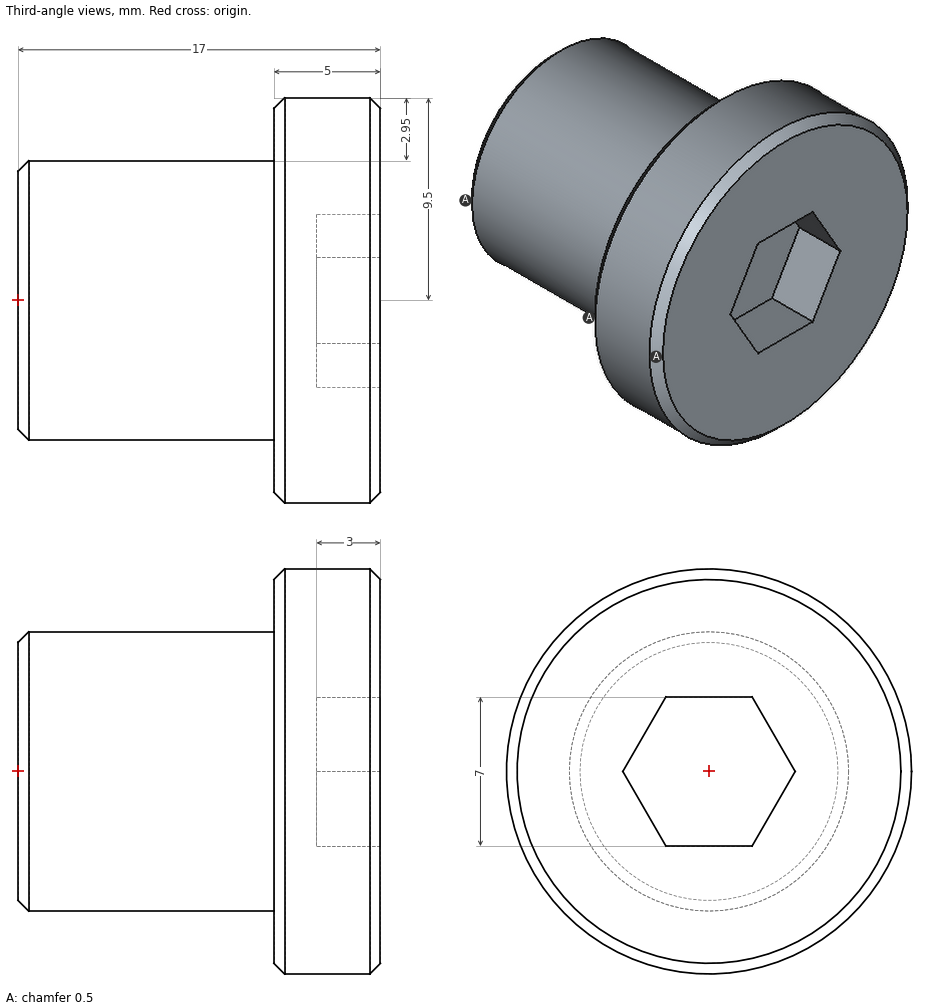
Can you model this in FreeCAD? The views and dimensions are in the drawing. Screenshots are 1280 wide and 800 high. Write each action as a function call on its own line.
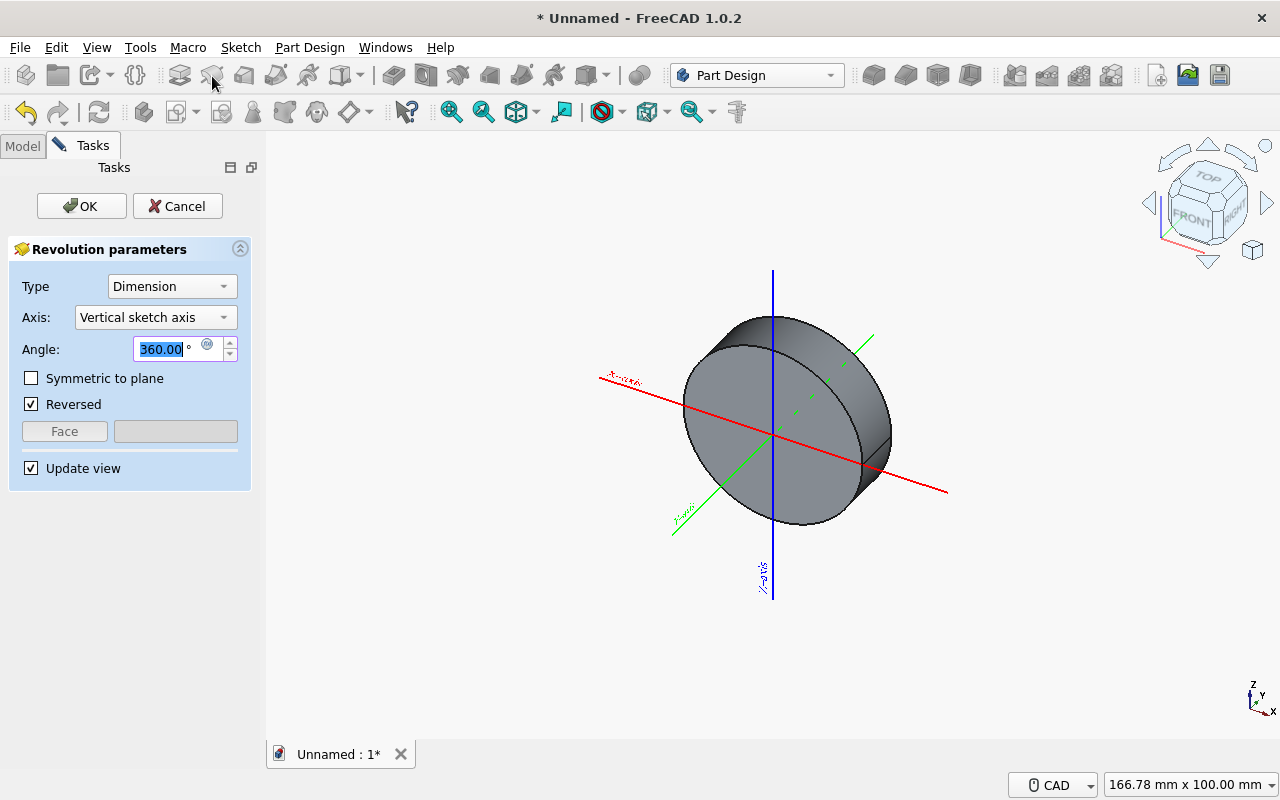
click(156, 318)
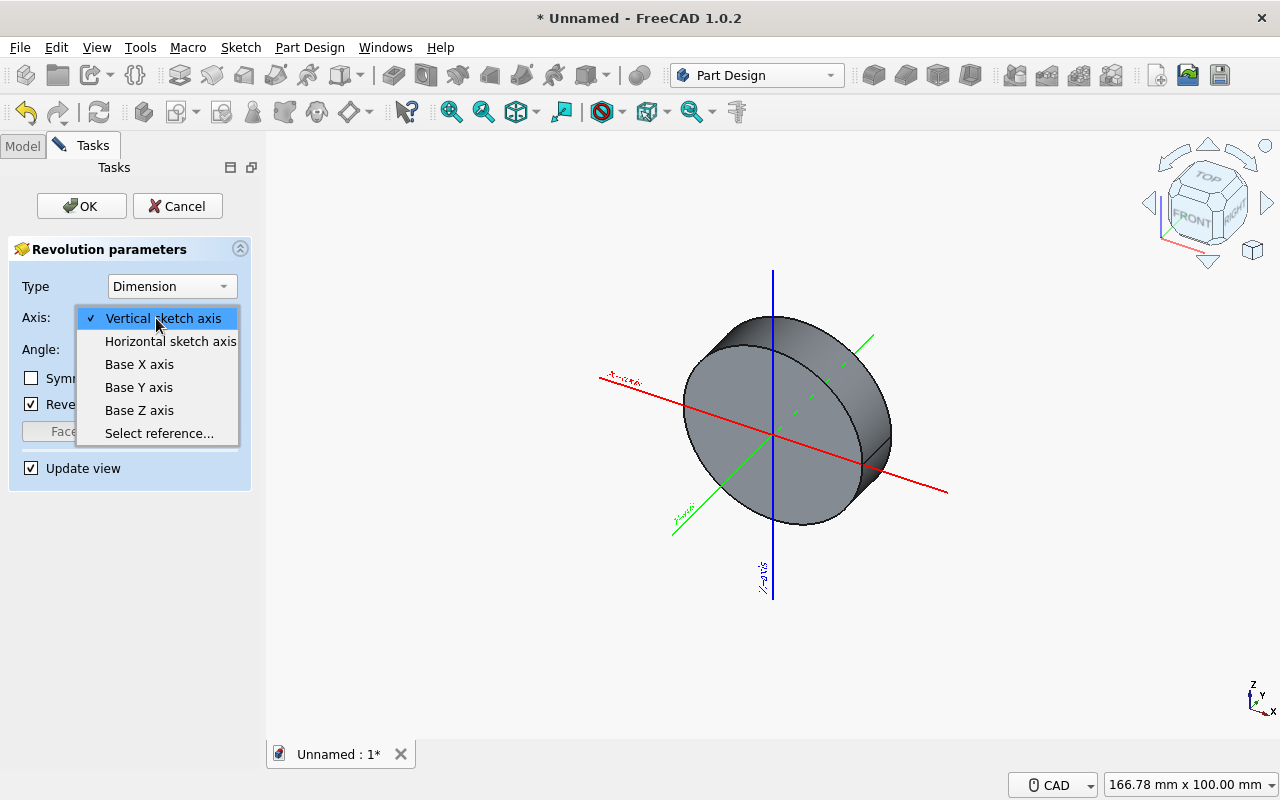
click(156, 342)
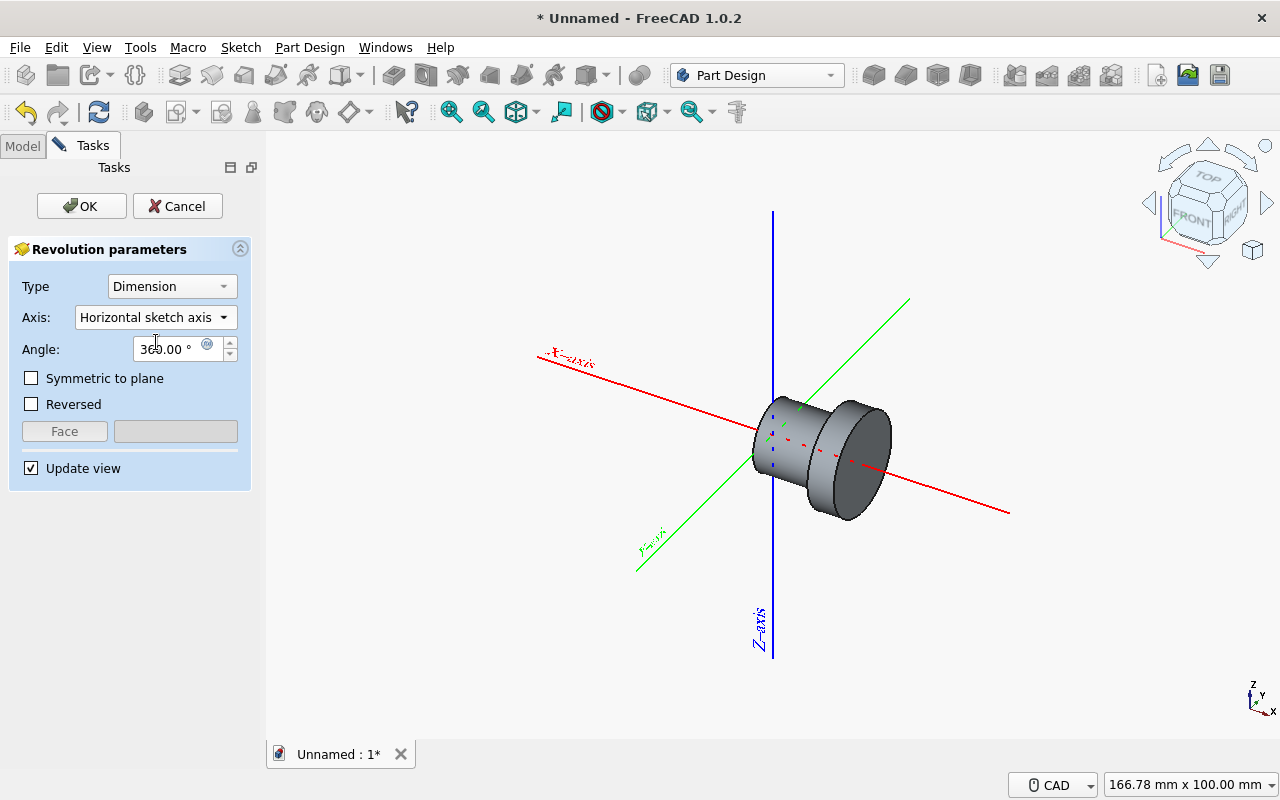
click(82, 206)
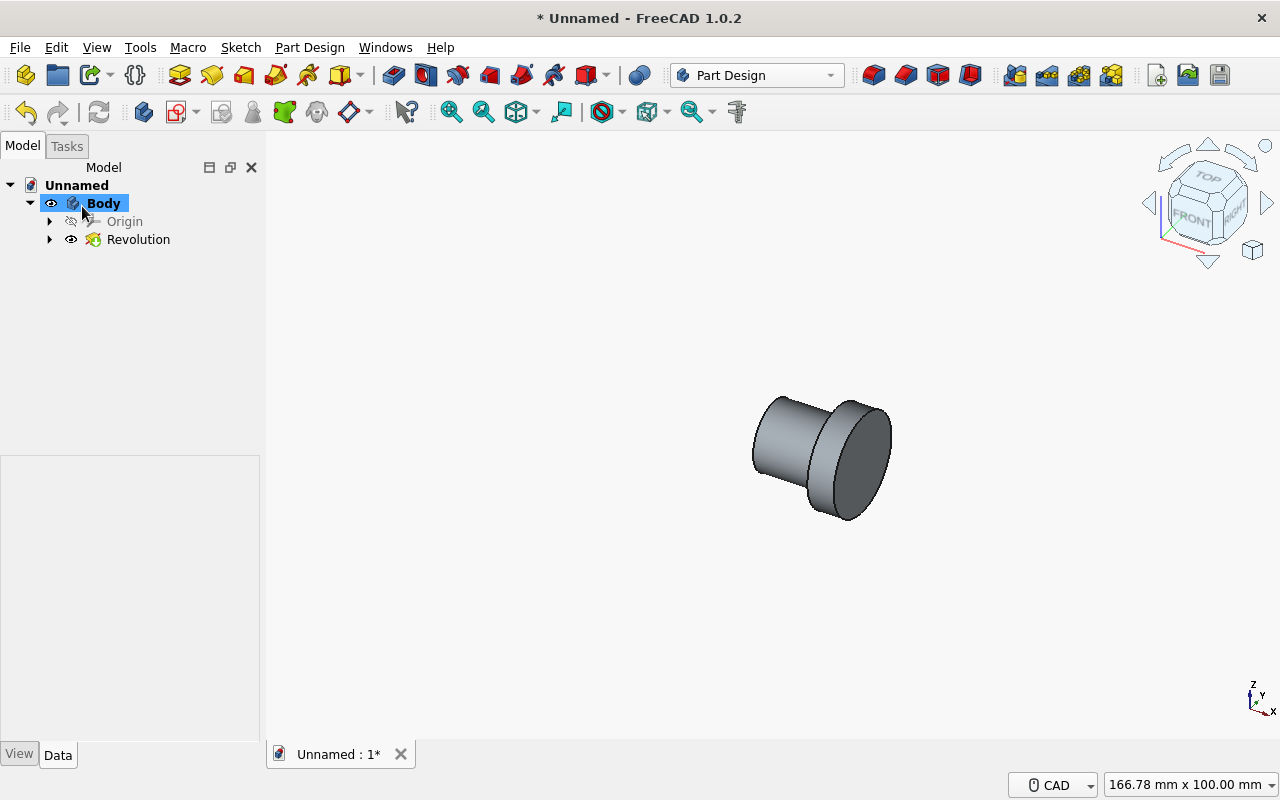
key(v)
key(f)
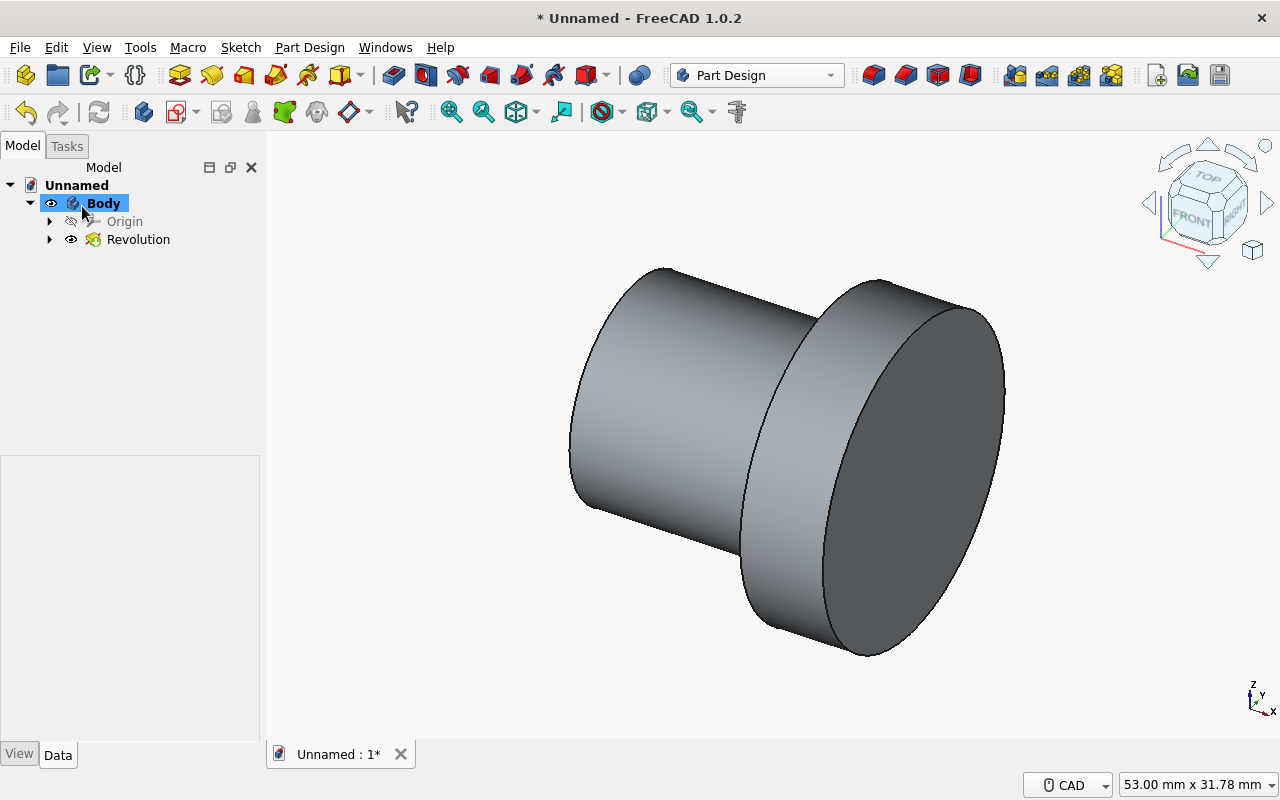
click(914, 481)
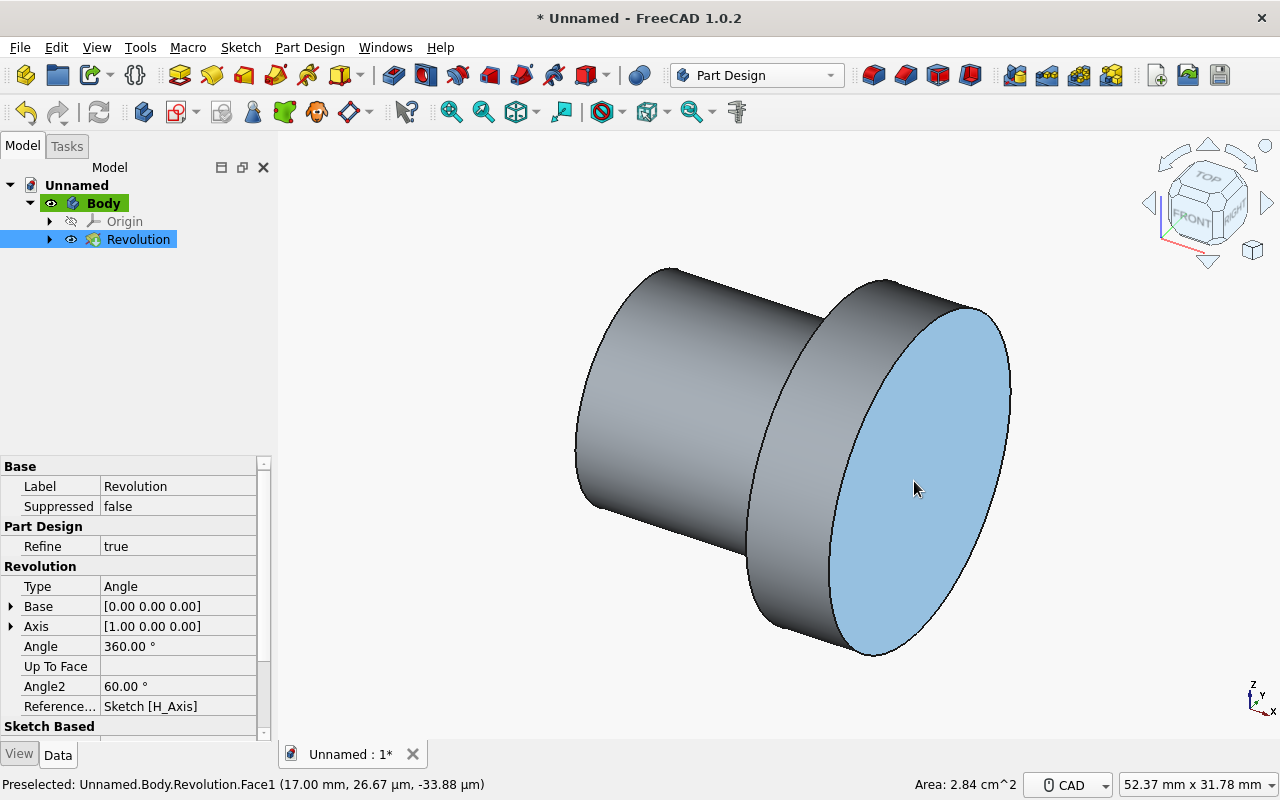
click(176, 112)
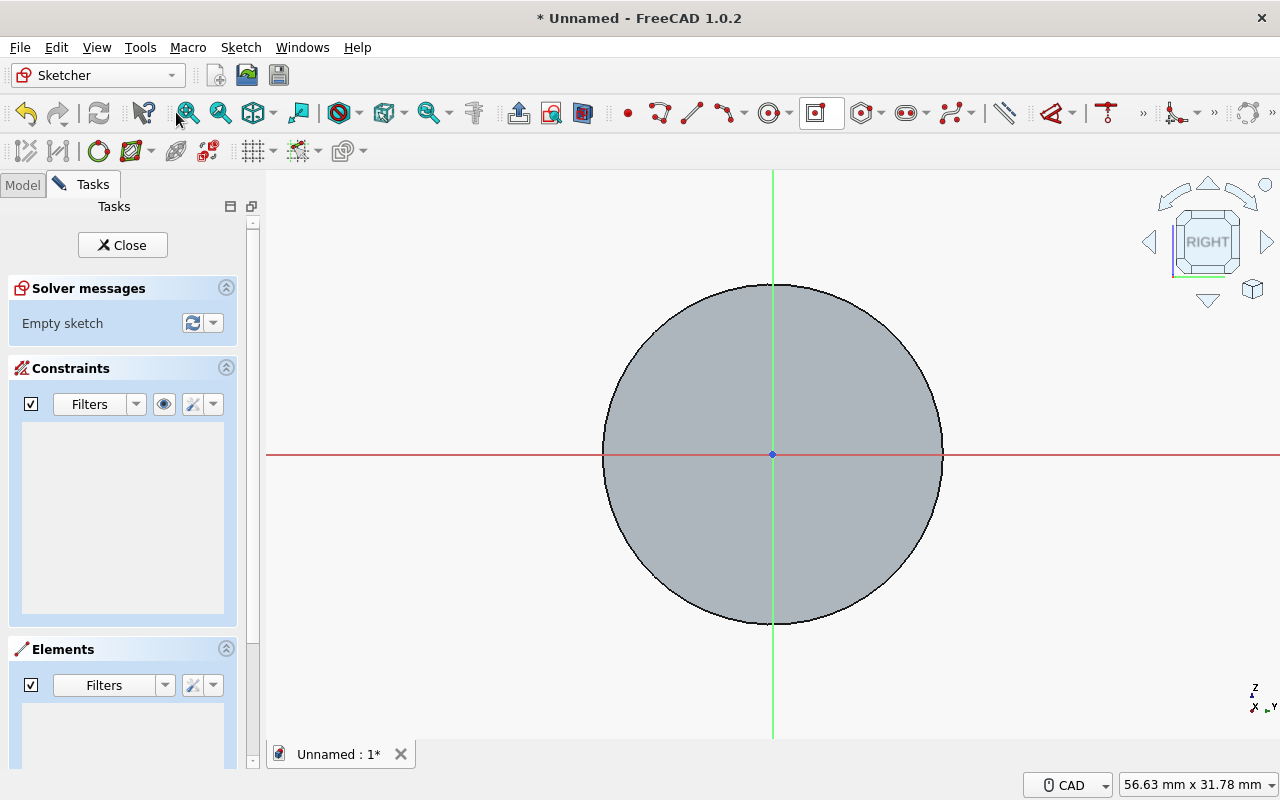
scroll(813, 454, up, 5)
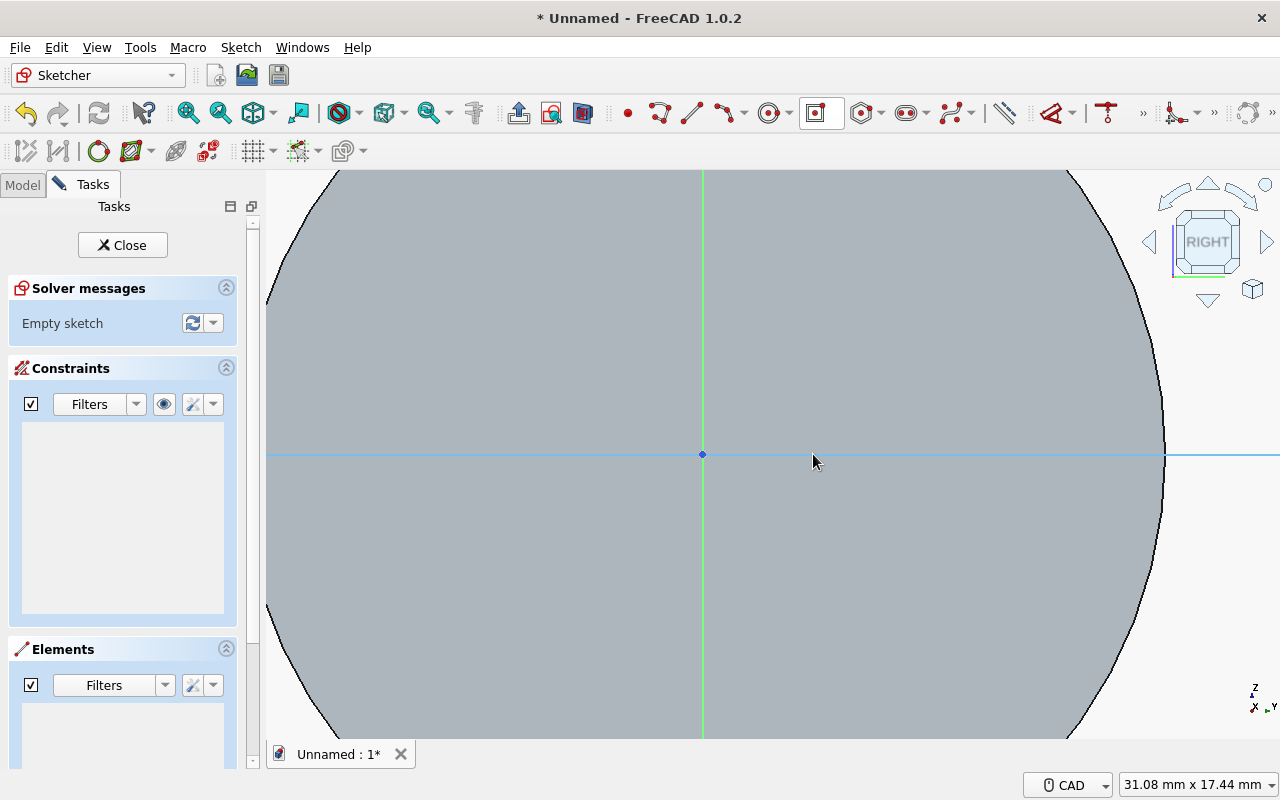
click(862, 114)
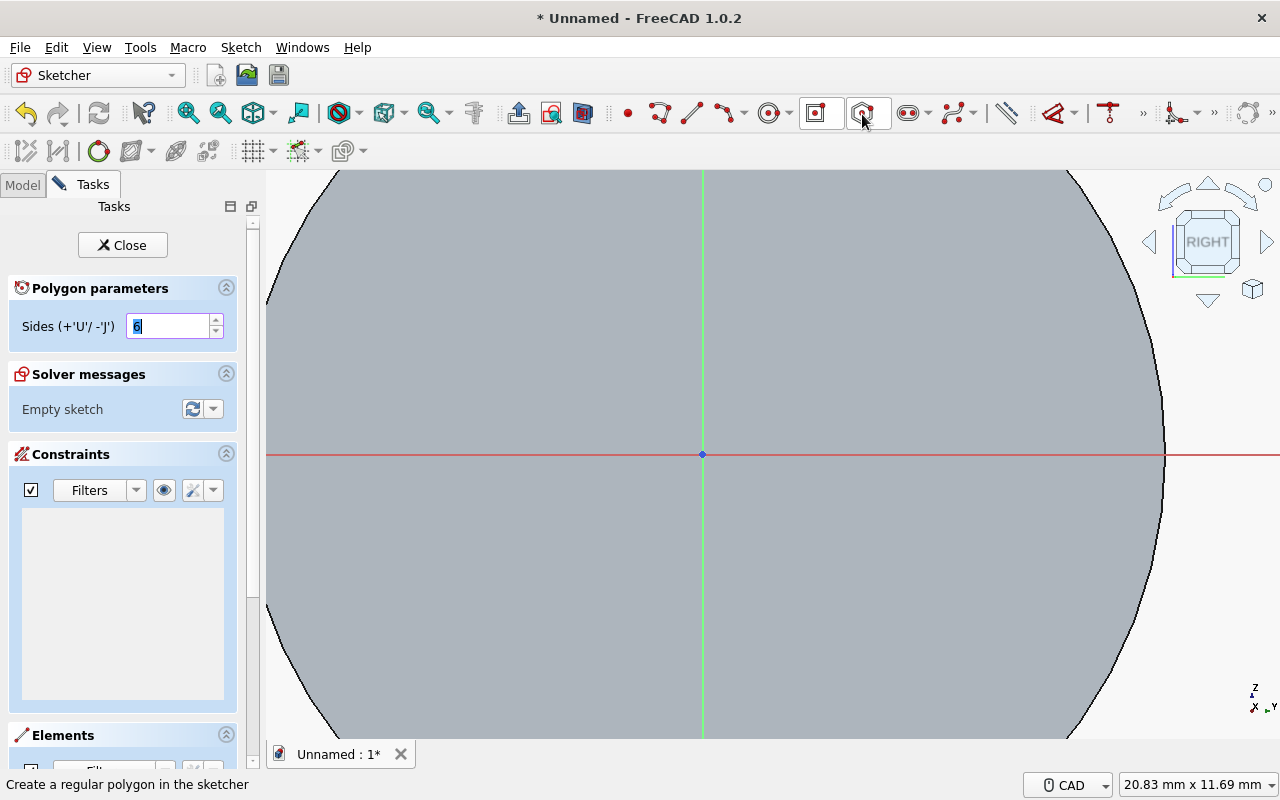
click(703, 454)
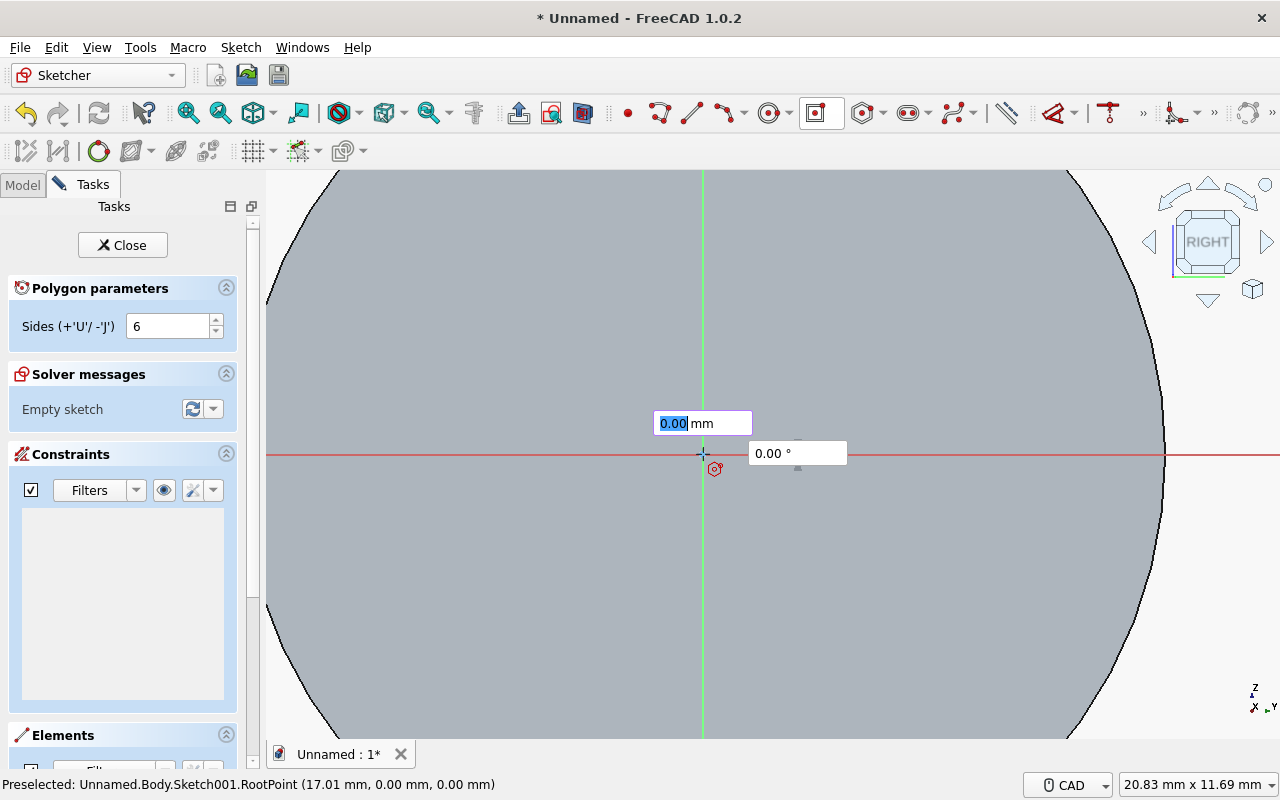
click(900, 454)
right_click(900, 454)